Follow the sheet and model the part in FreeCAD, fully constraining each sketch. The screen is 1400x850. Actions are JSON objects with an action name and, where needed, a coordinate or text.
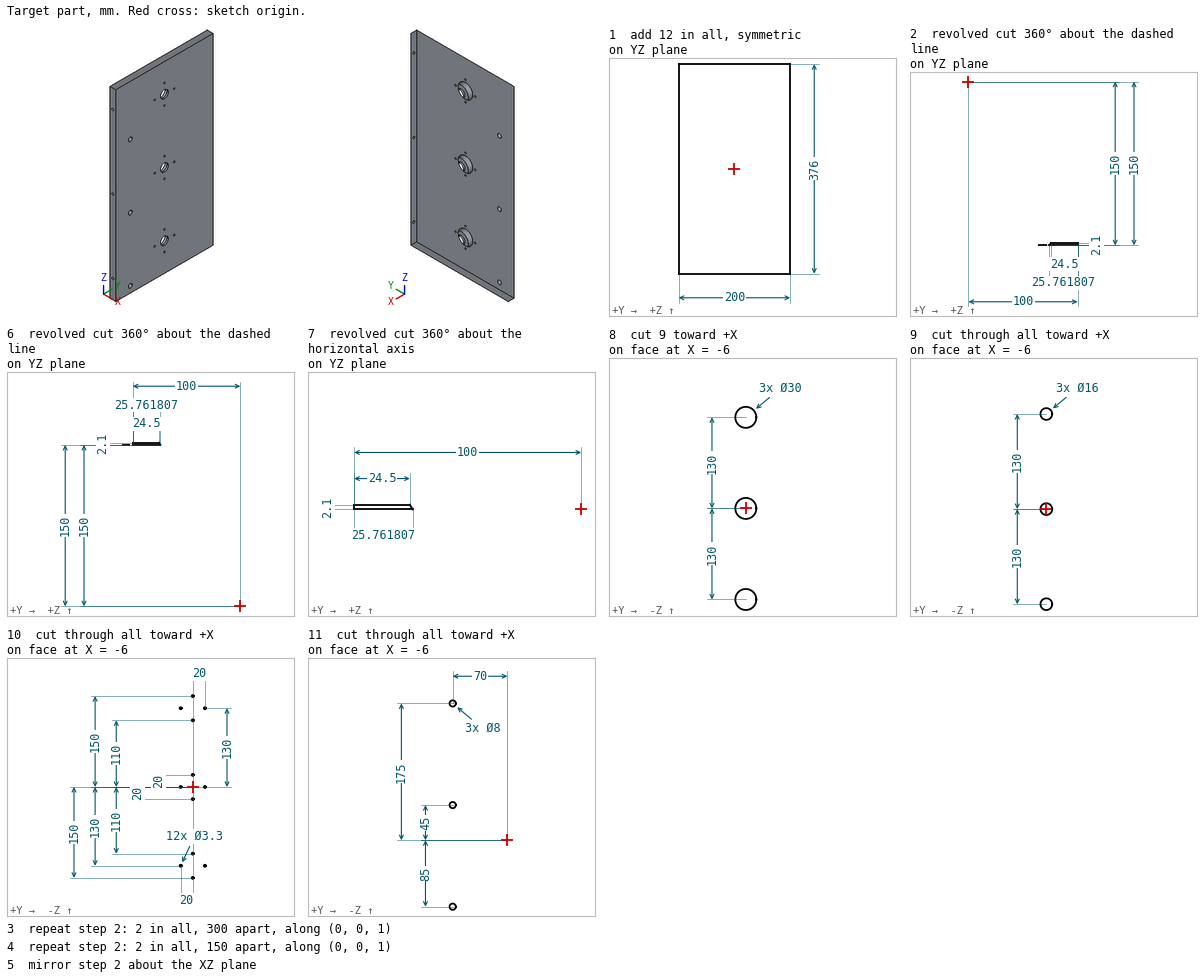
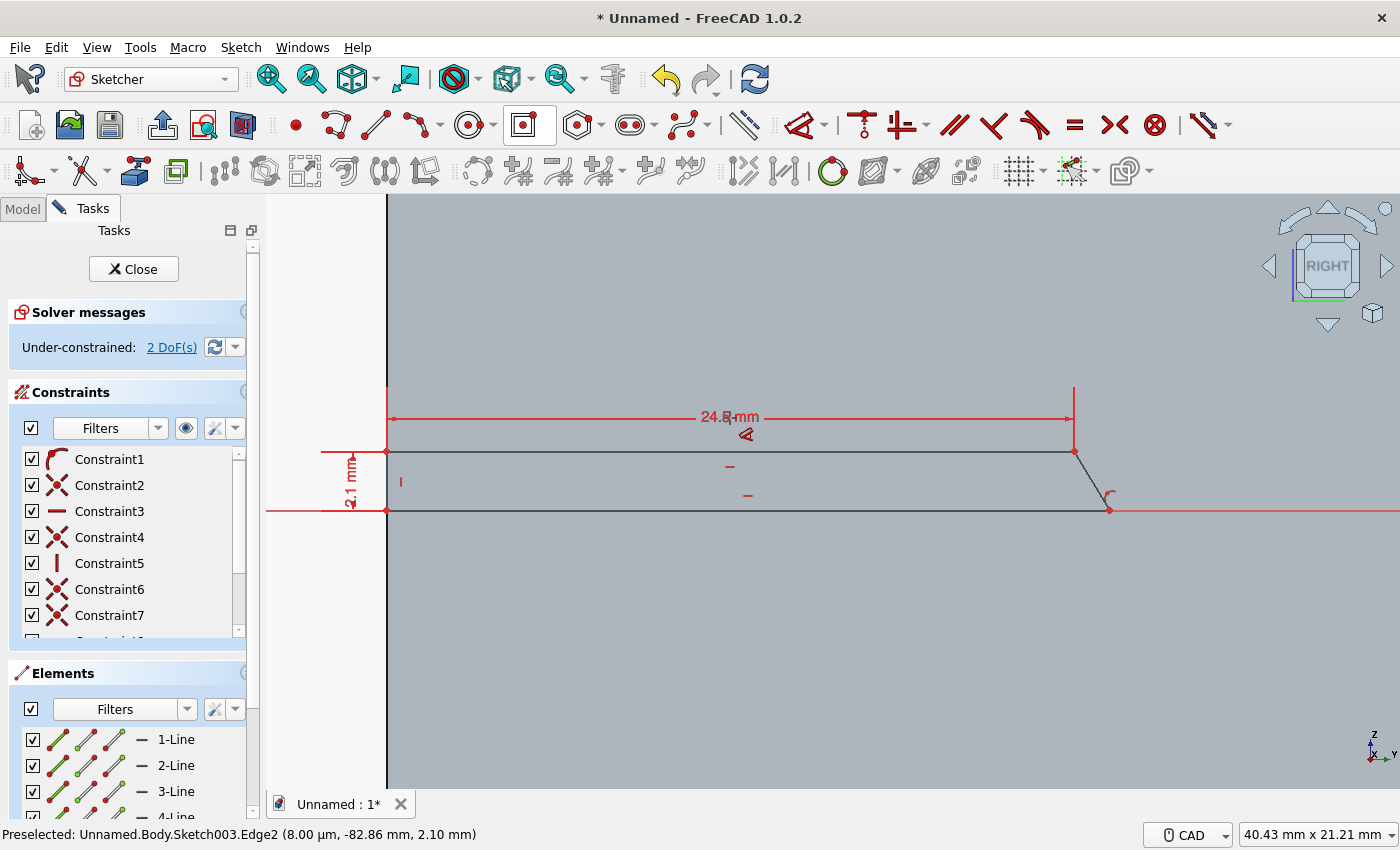
{"action": "left_click", "coordinate": [387, 452]}
{"action": "left_click", "coordinate": [811, 545]}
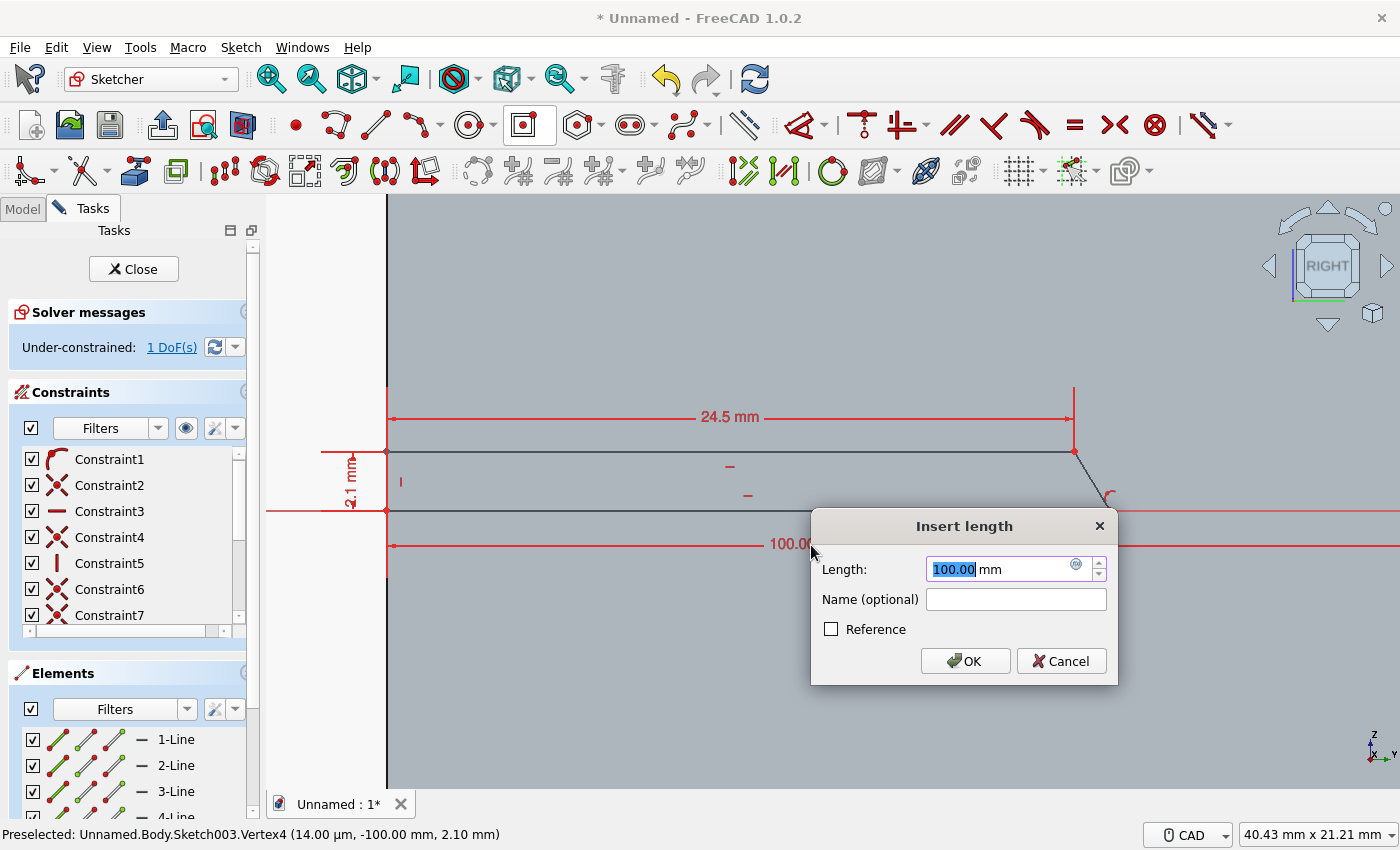
{"action": "type", "text": "100"}
{"action": "key", "text": "Return"}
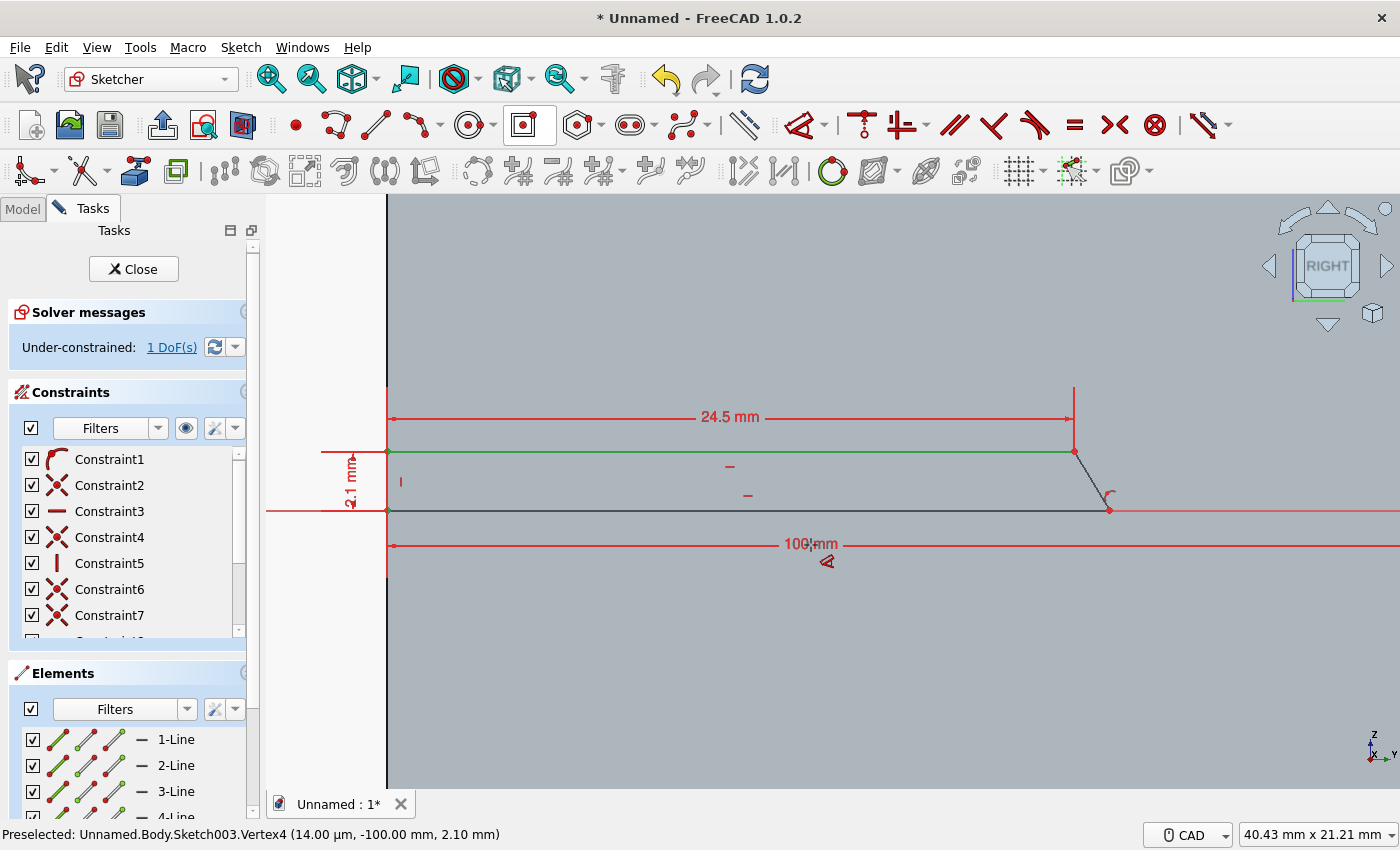
{"action": "left_click", "coordinate": [604, 511]}
{"action": "left_click", "coordinate": [582, 545]}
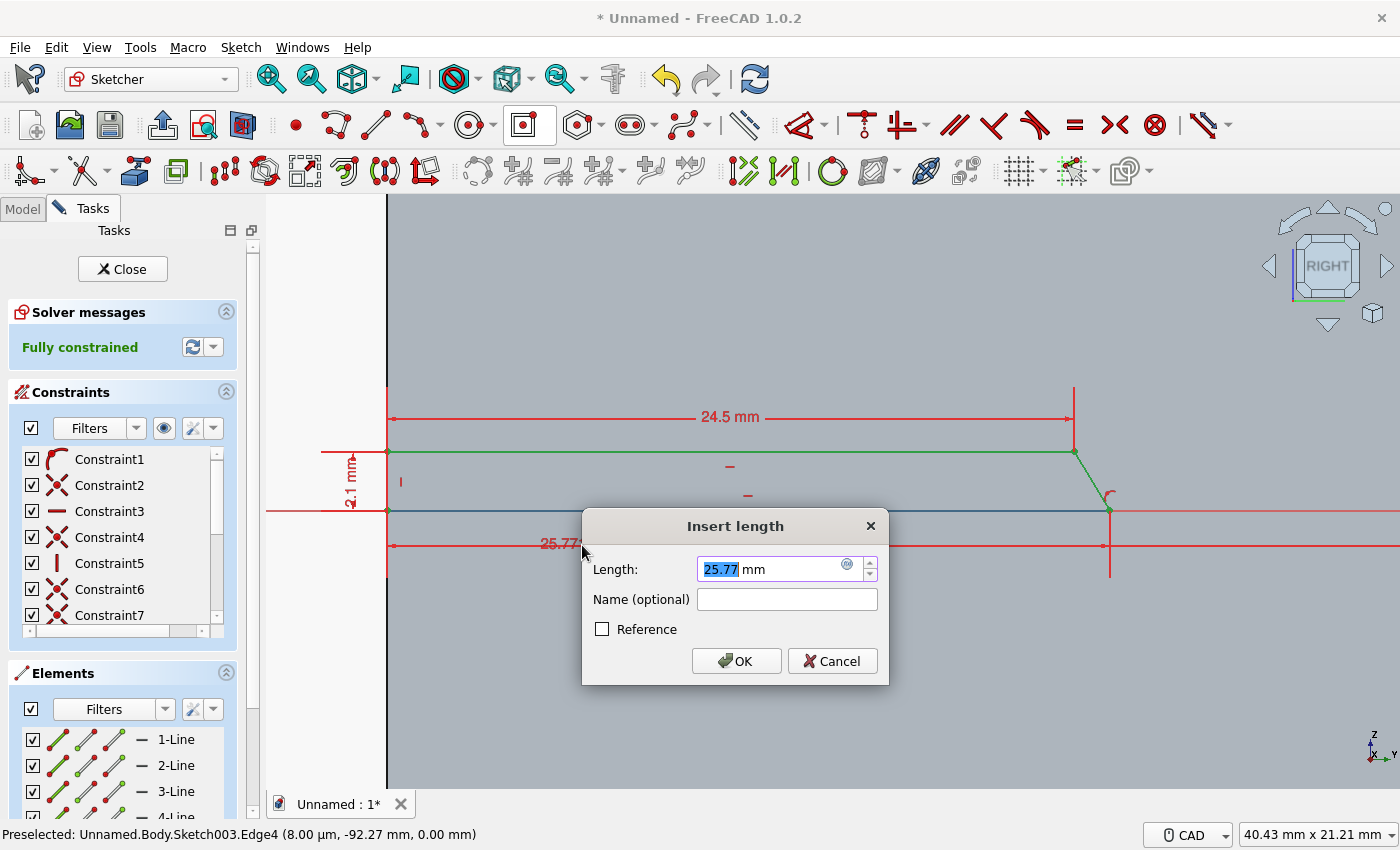
{"action": "type", "text": "25.761807"}
{"action": "key", "text": "Return"}
{"action": "key", "text": "Escape"}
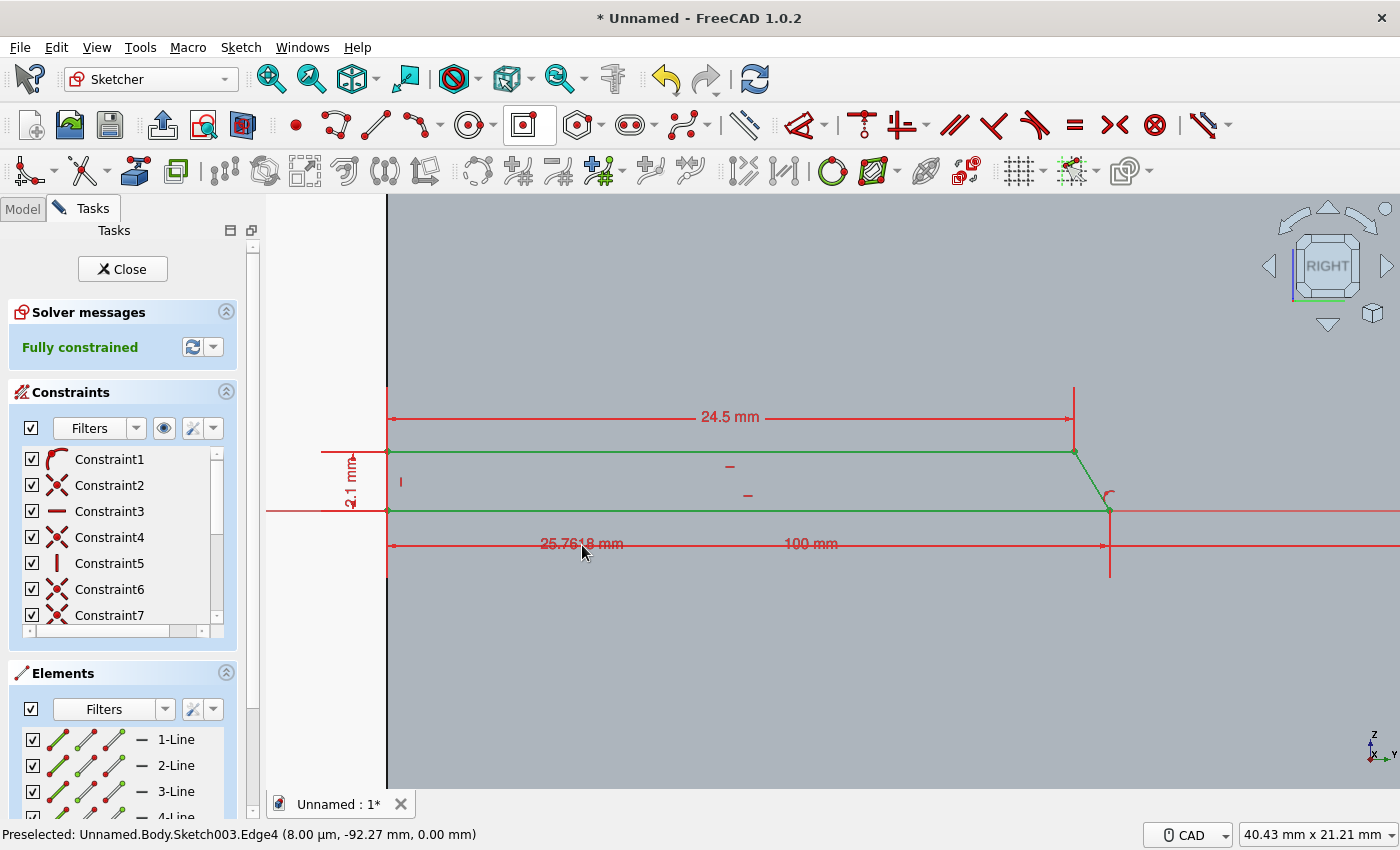
{"action": "left_click", "coordinate": [123, 269]}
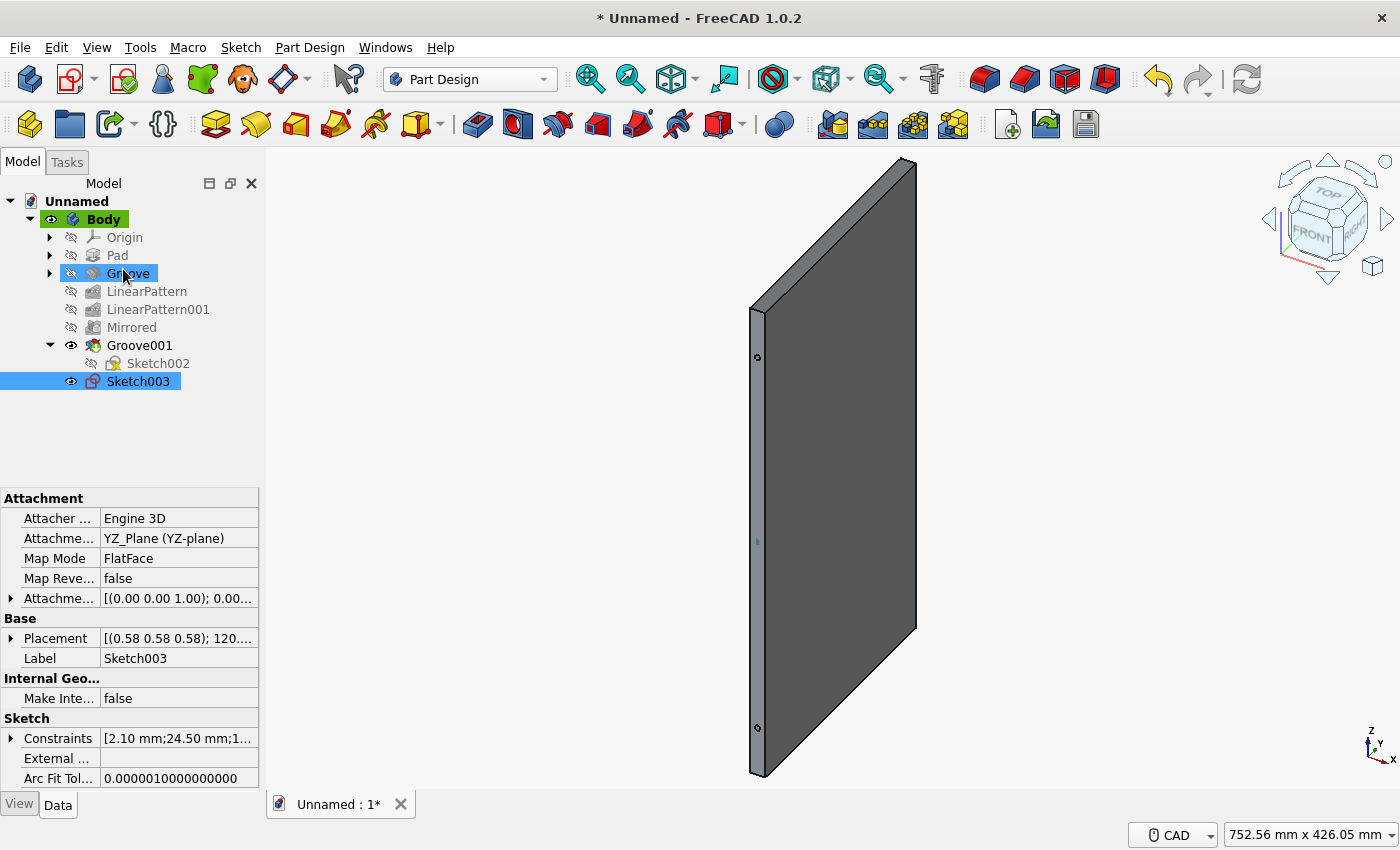
{"action": "left_click", "coordinate": [558, 124]}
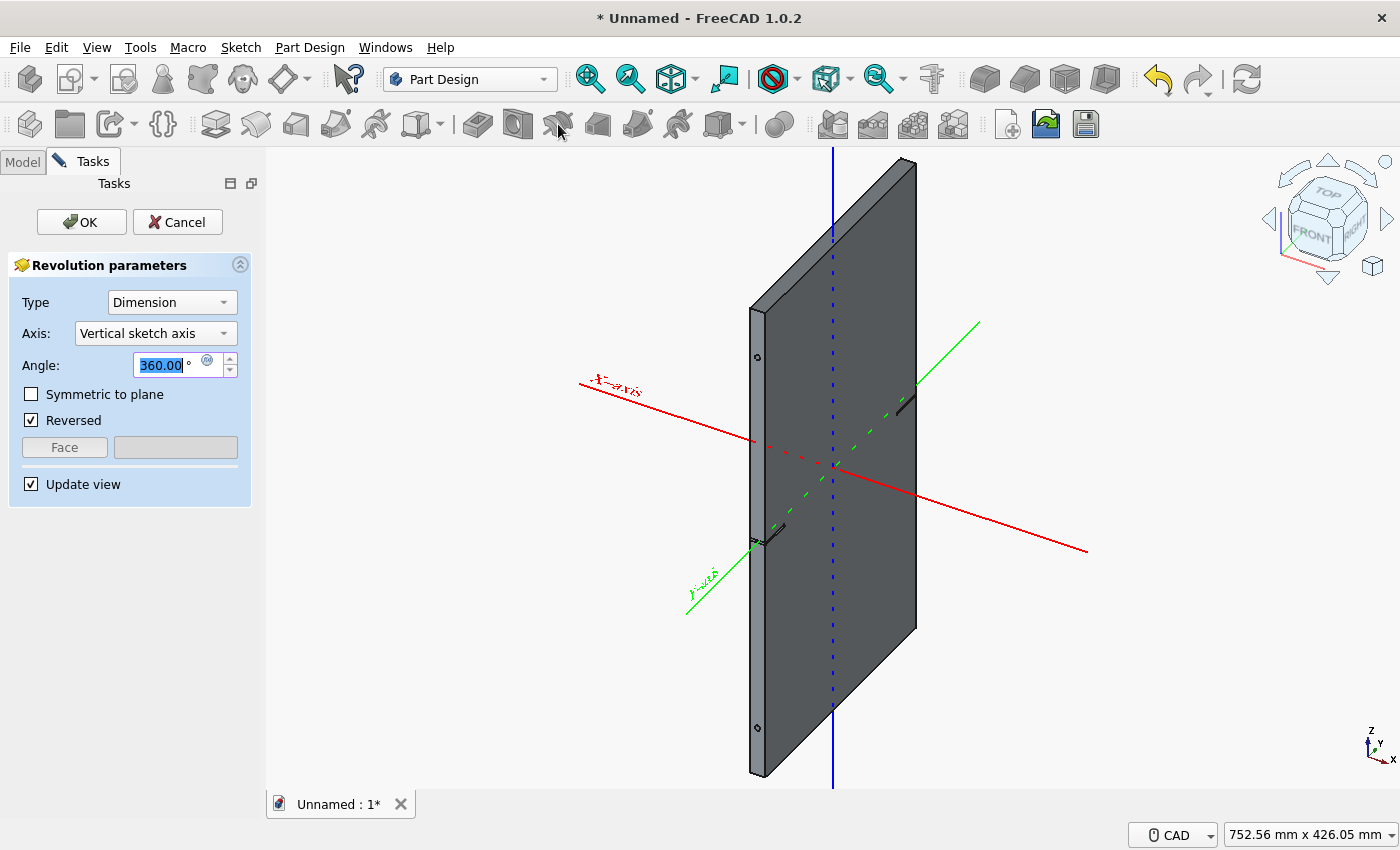
{"action": "left_click", "coordinate": [156, 334]}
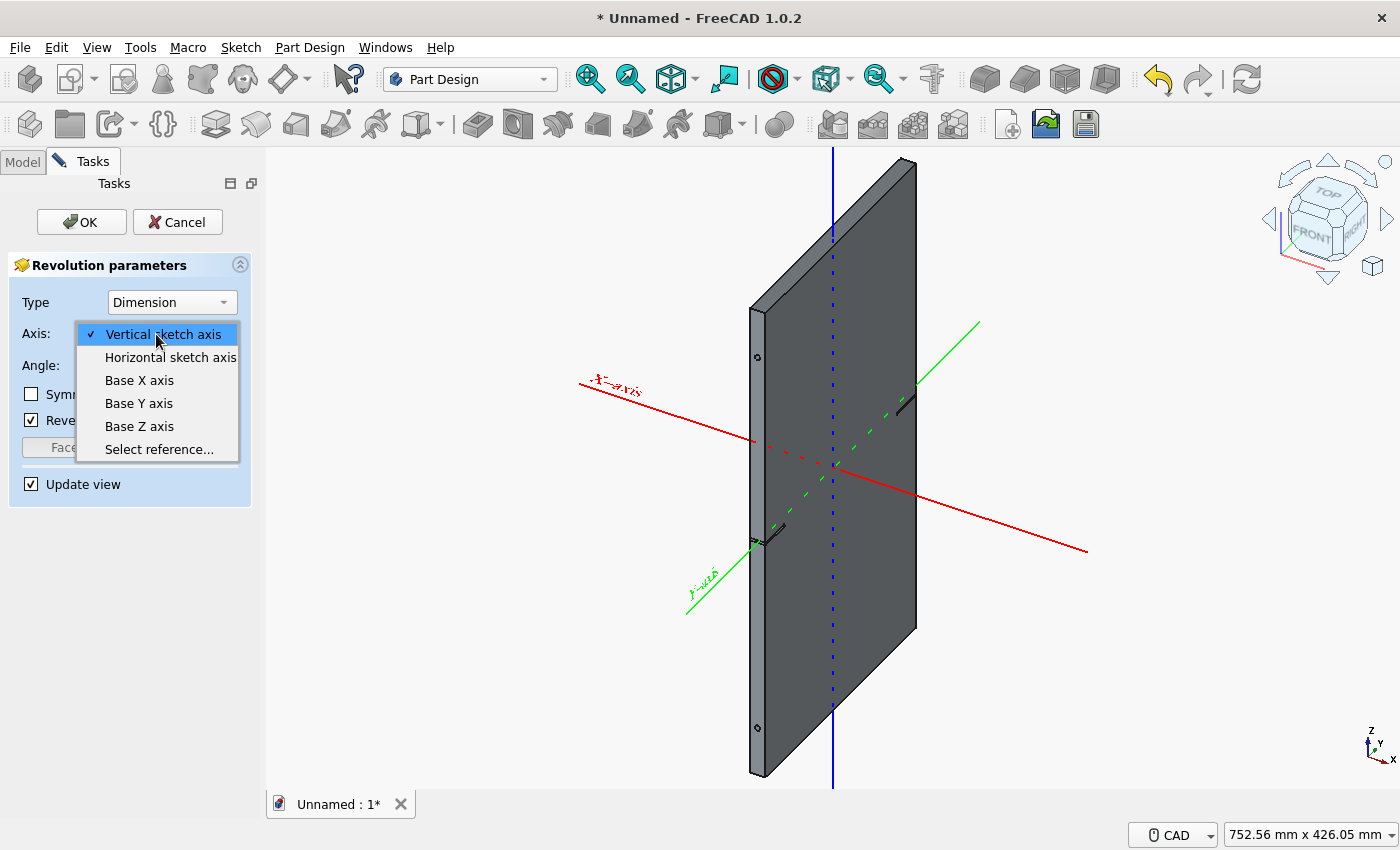
{"action": "left_click", "coordinate": [156, 358]}